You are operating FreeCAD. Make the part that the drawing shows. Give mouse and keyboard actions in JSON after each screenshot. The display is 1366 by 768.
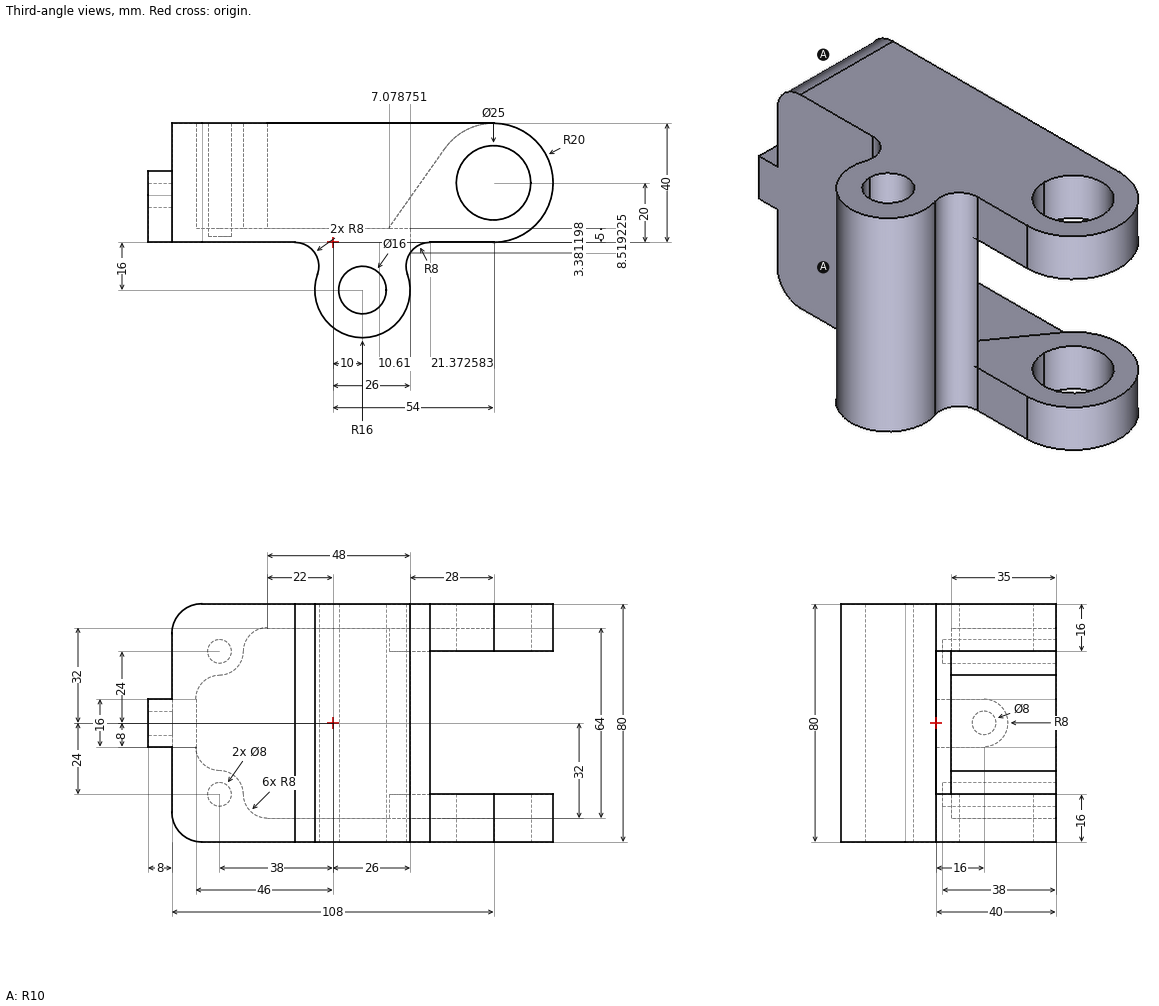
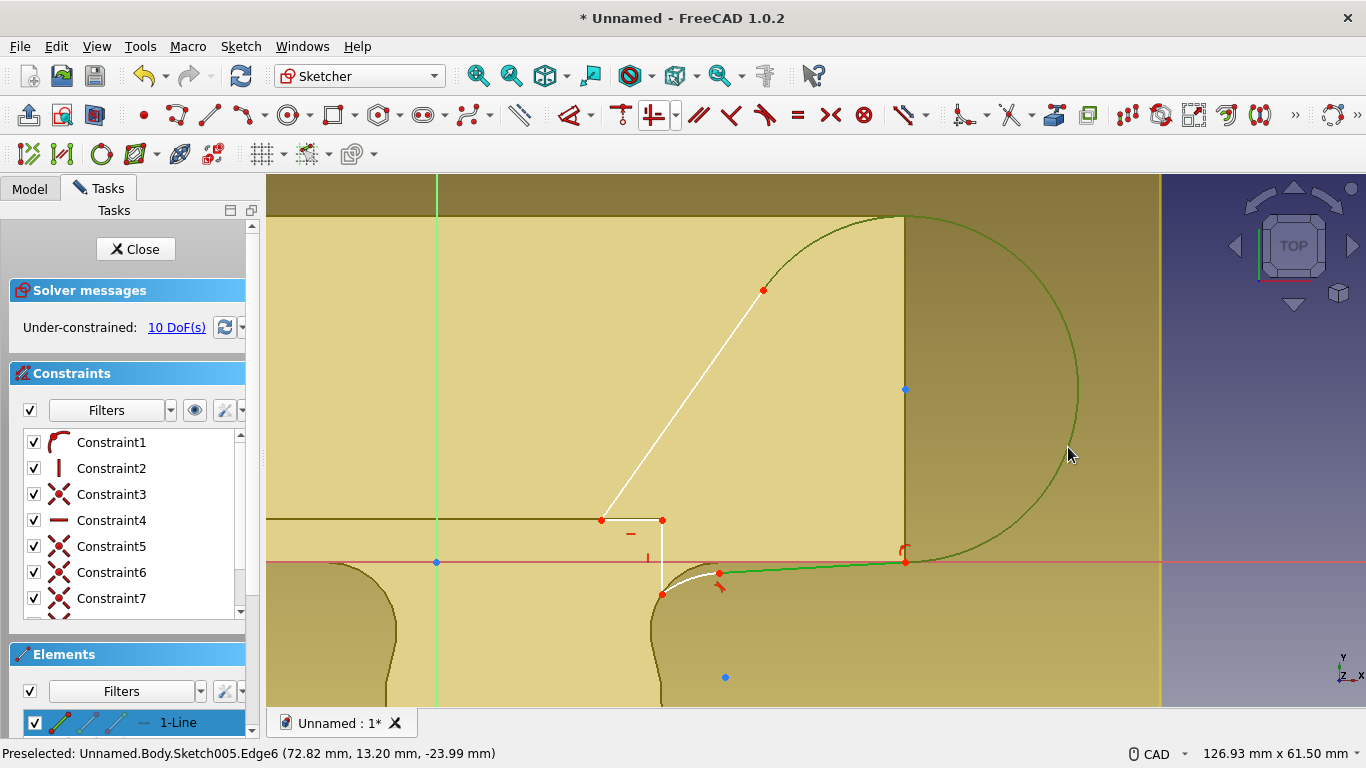
{"action": "key", "text": "t"}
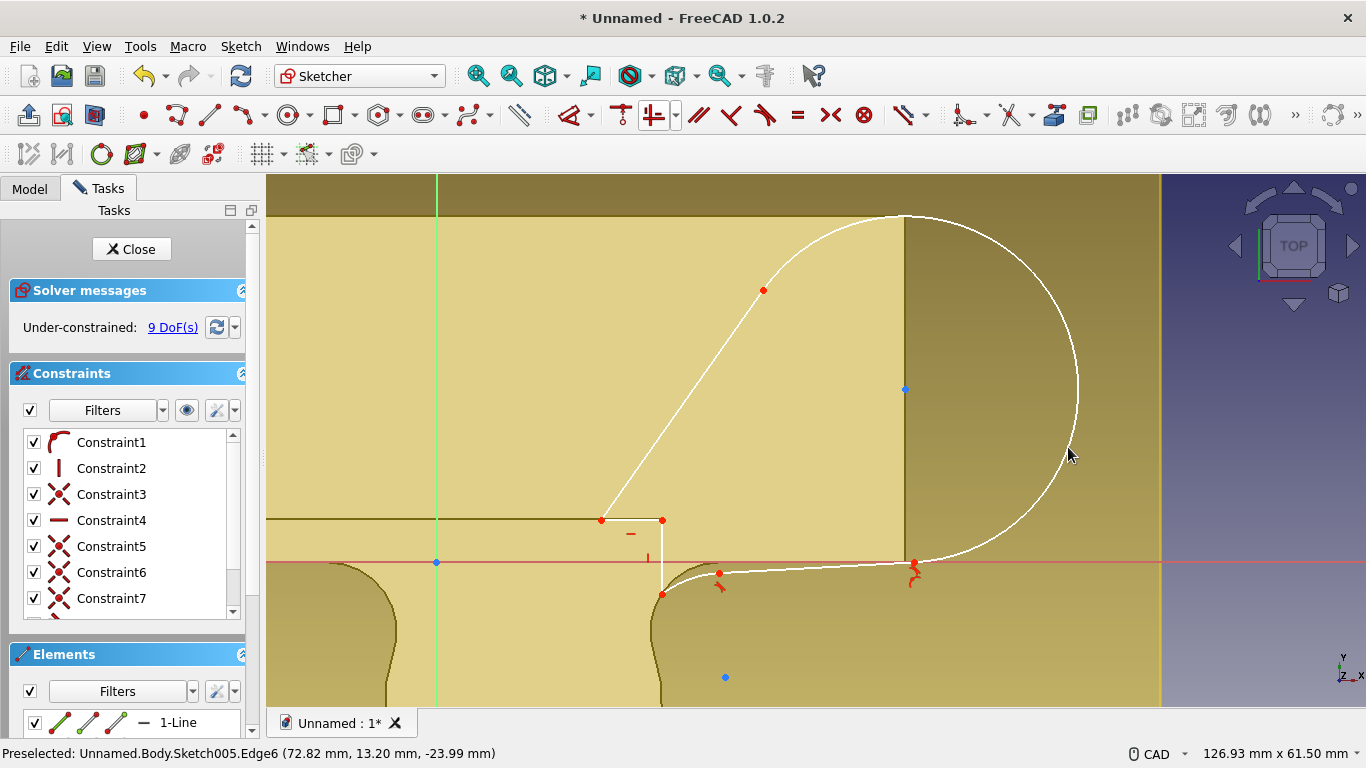
{"action": "left_click", "coordinate": [650, 451]}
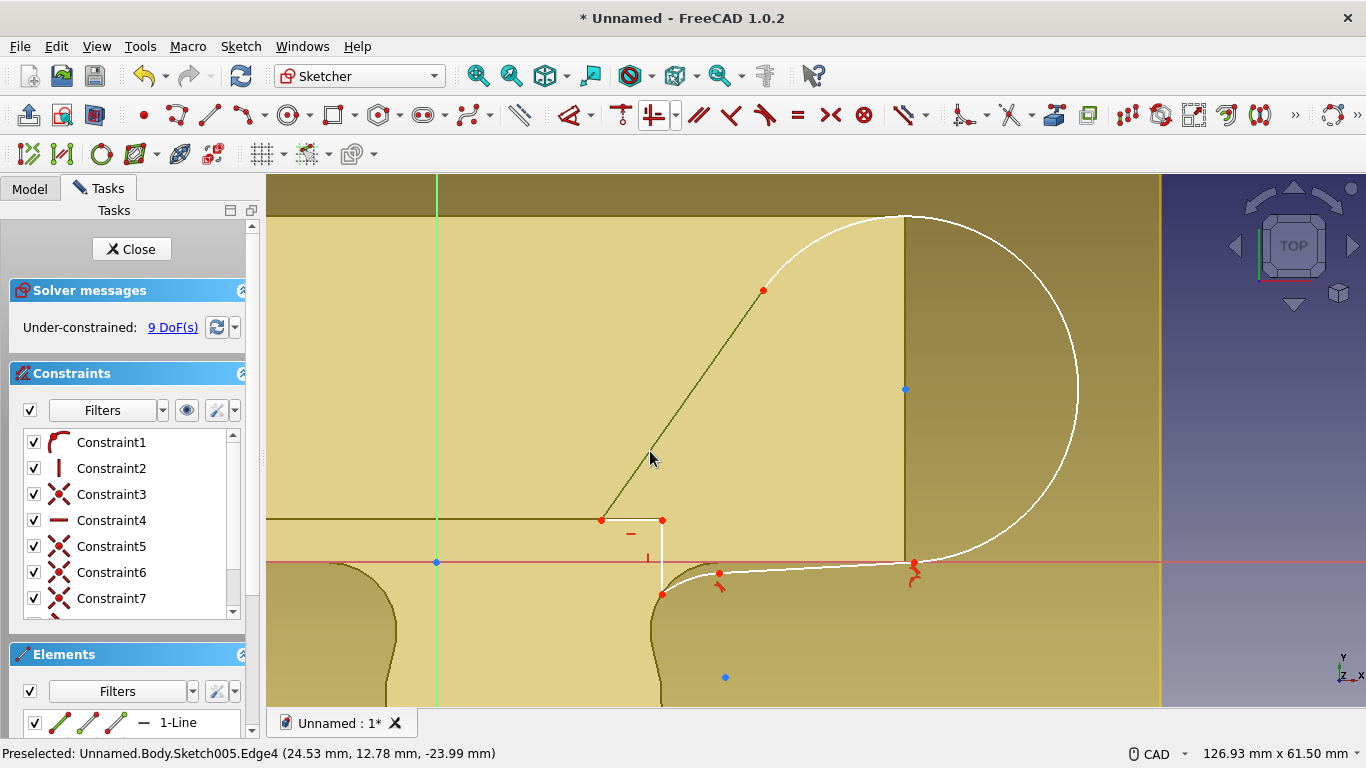
{"action": "left_click", "coordinate": [1070, 441]}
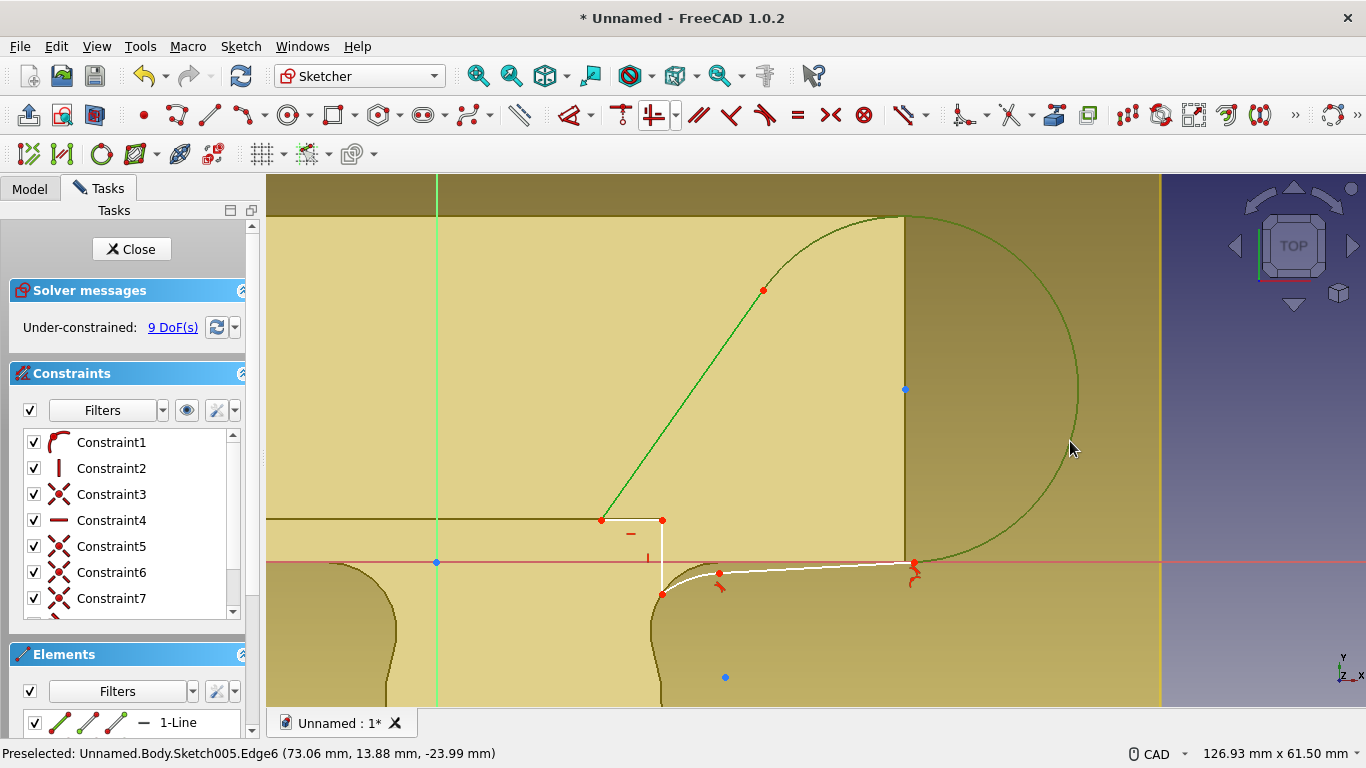
{"action": "key", "text": "t"}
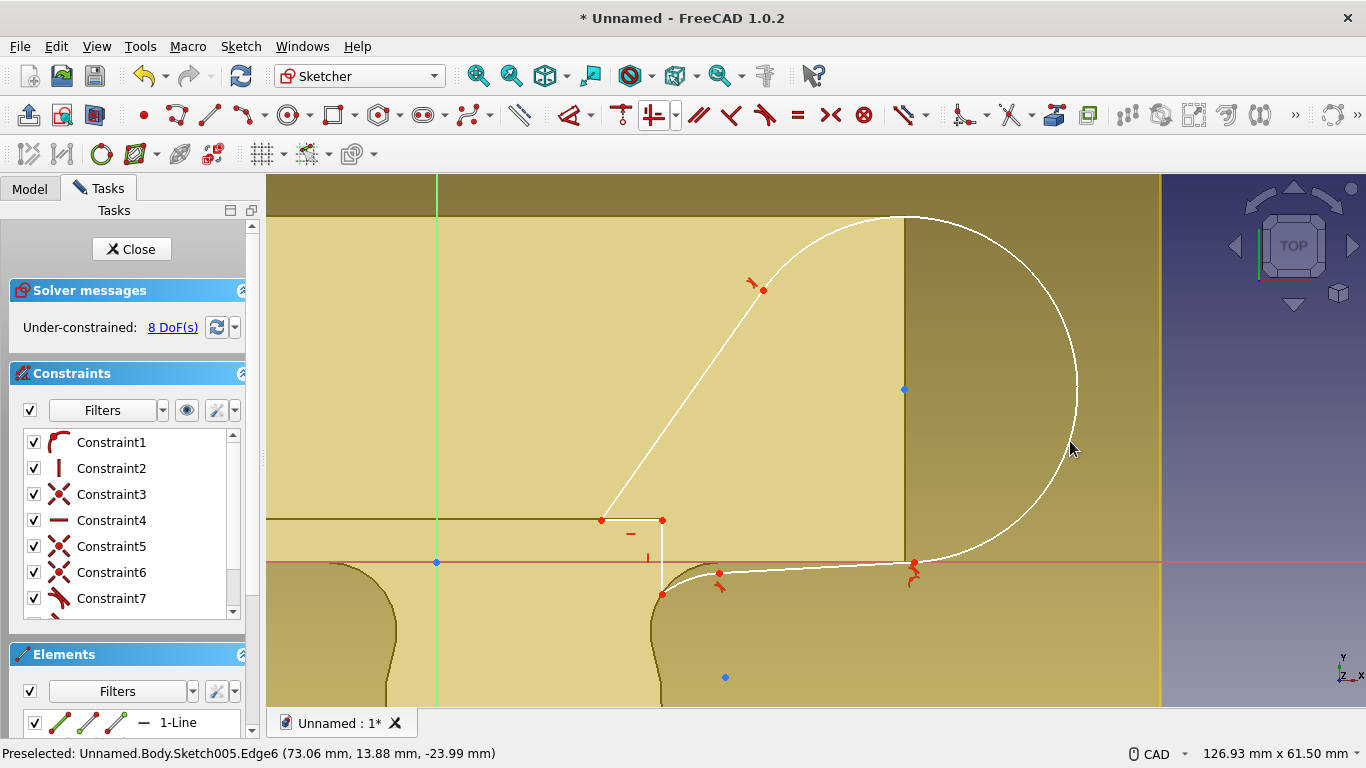
{"action": "left_click", "coordinate": [856, 566]}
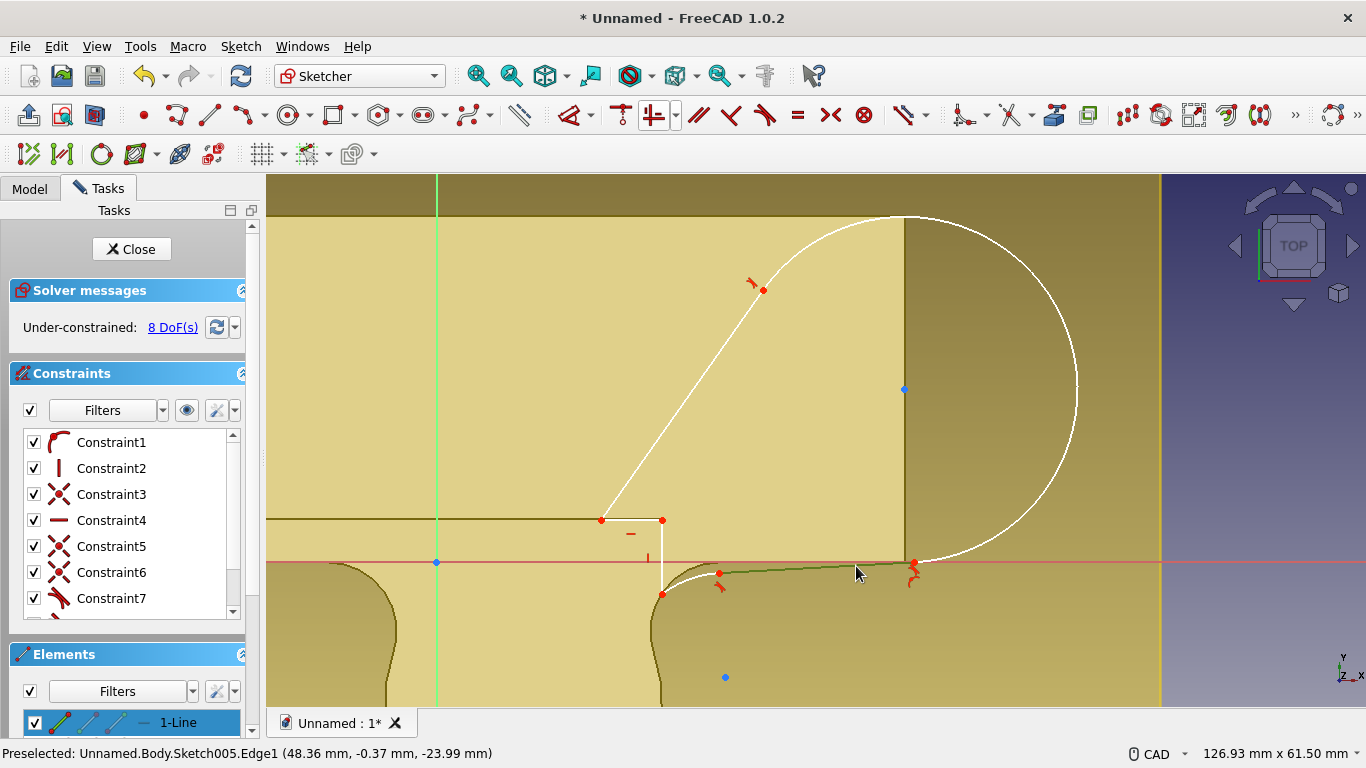
{"action": "key", "text": "h"}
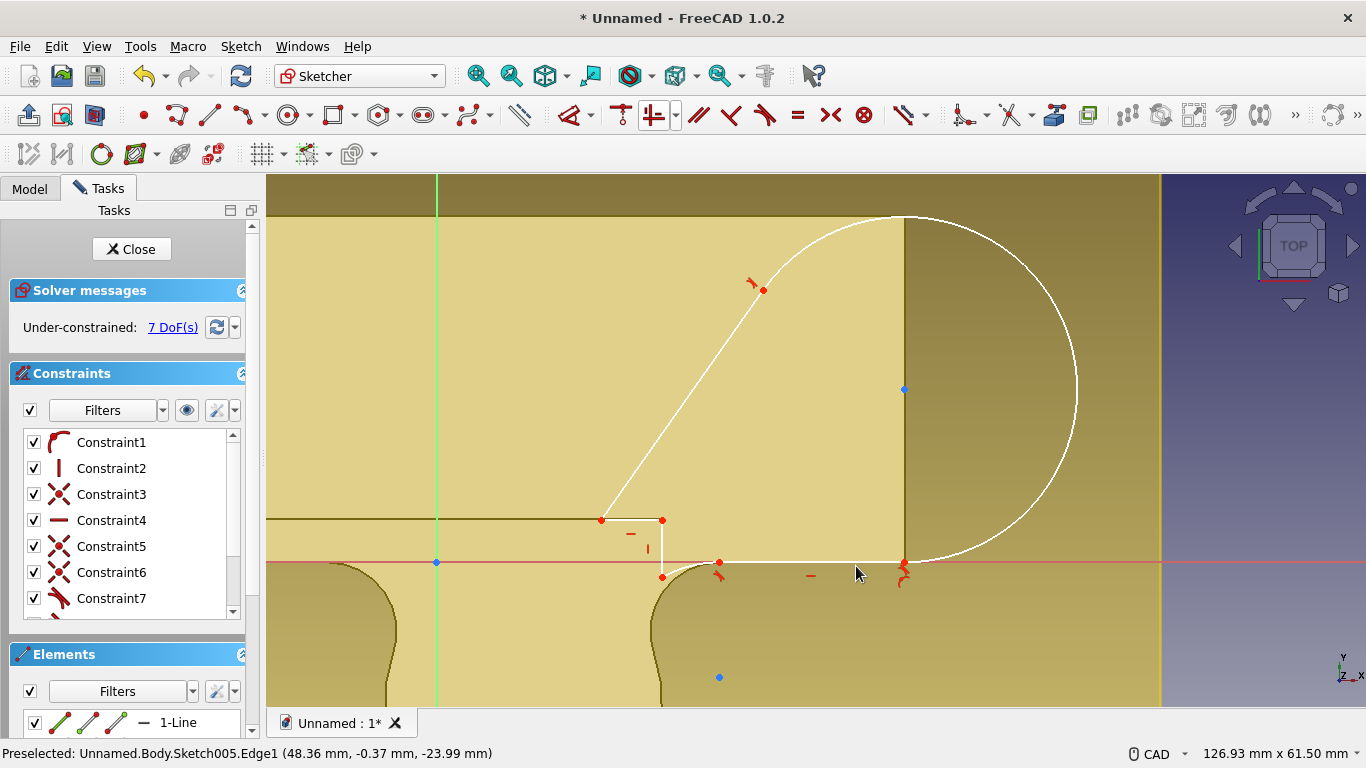
{"action": "key", "text": "d"}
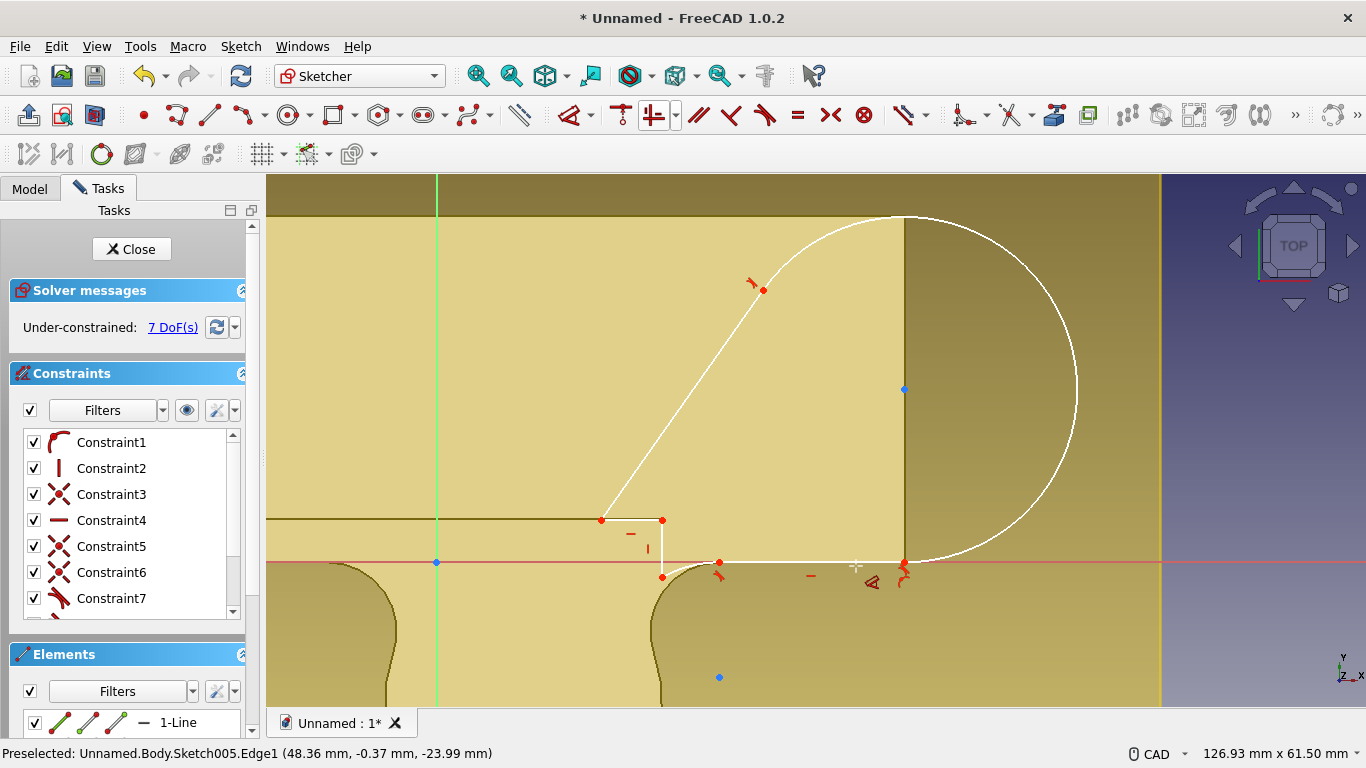
{"action": "left_click", "coordinate": [701, 564]}
{"action": "left_click", "coordinate": [696, 532]}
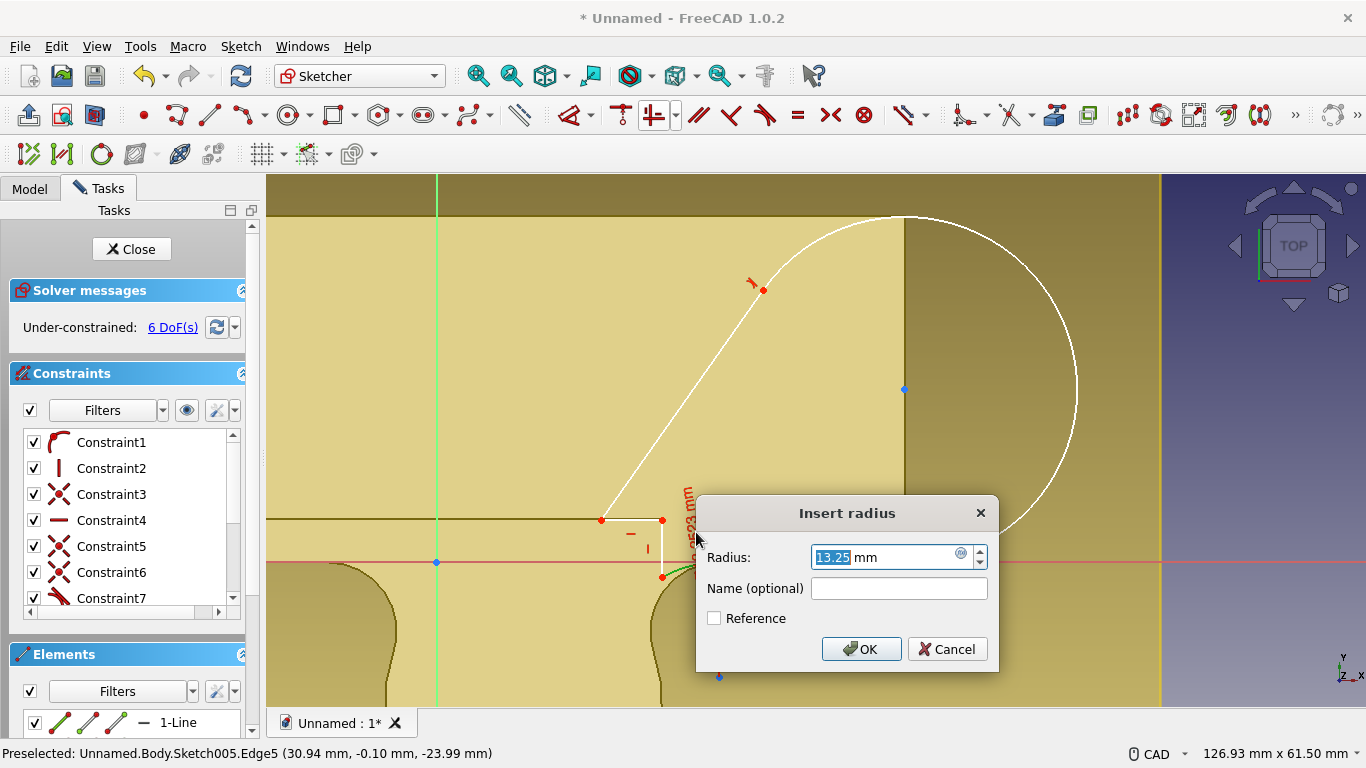
{"action": "type", "text": "8"}
{"action": "key", "text": "Return"}